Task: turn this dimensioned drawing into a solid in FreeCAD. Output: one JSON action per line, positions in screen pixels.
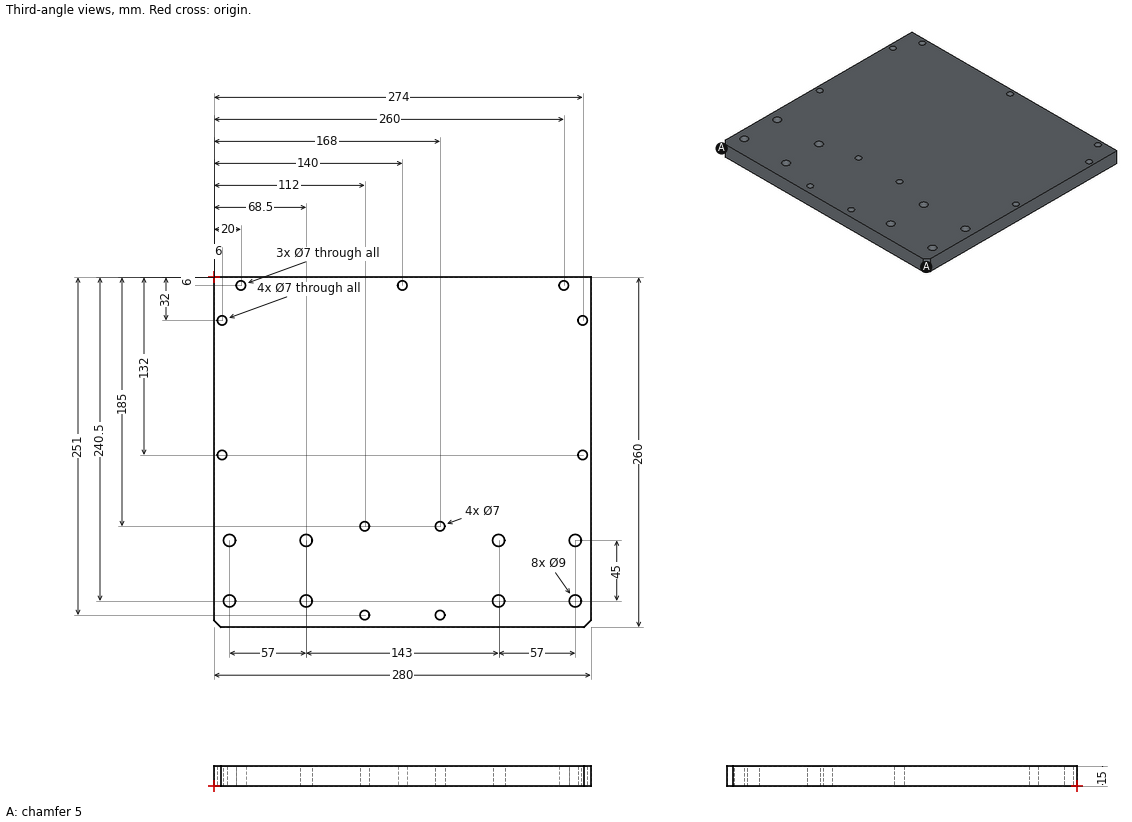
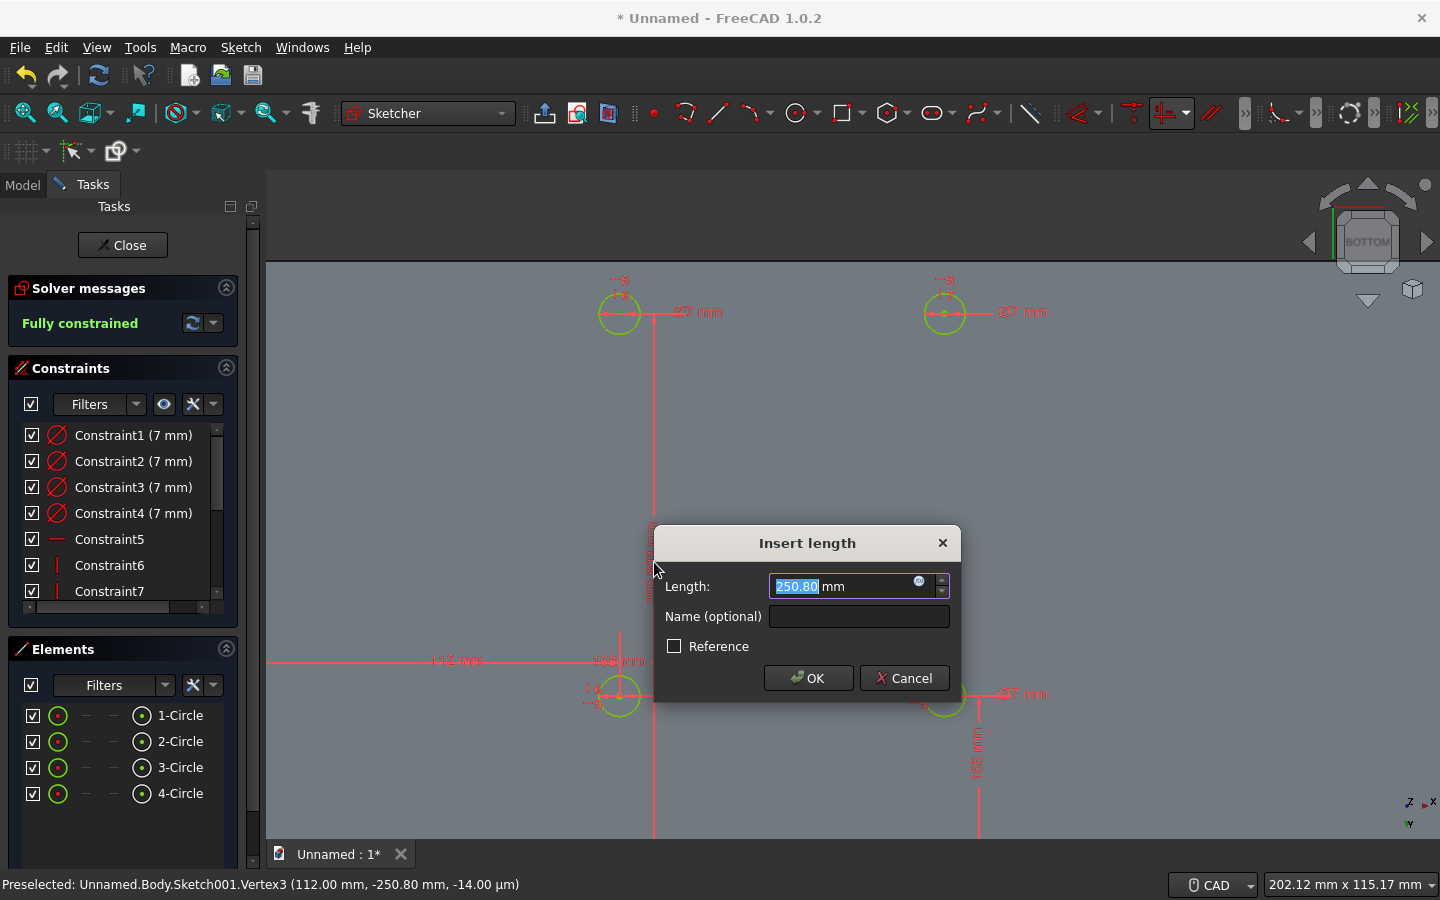
{"action": "type", "text": "251"}
{"action": "key", "text": "Return"}
{"action": "key", "text": "Escape"}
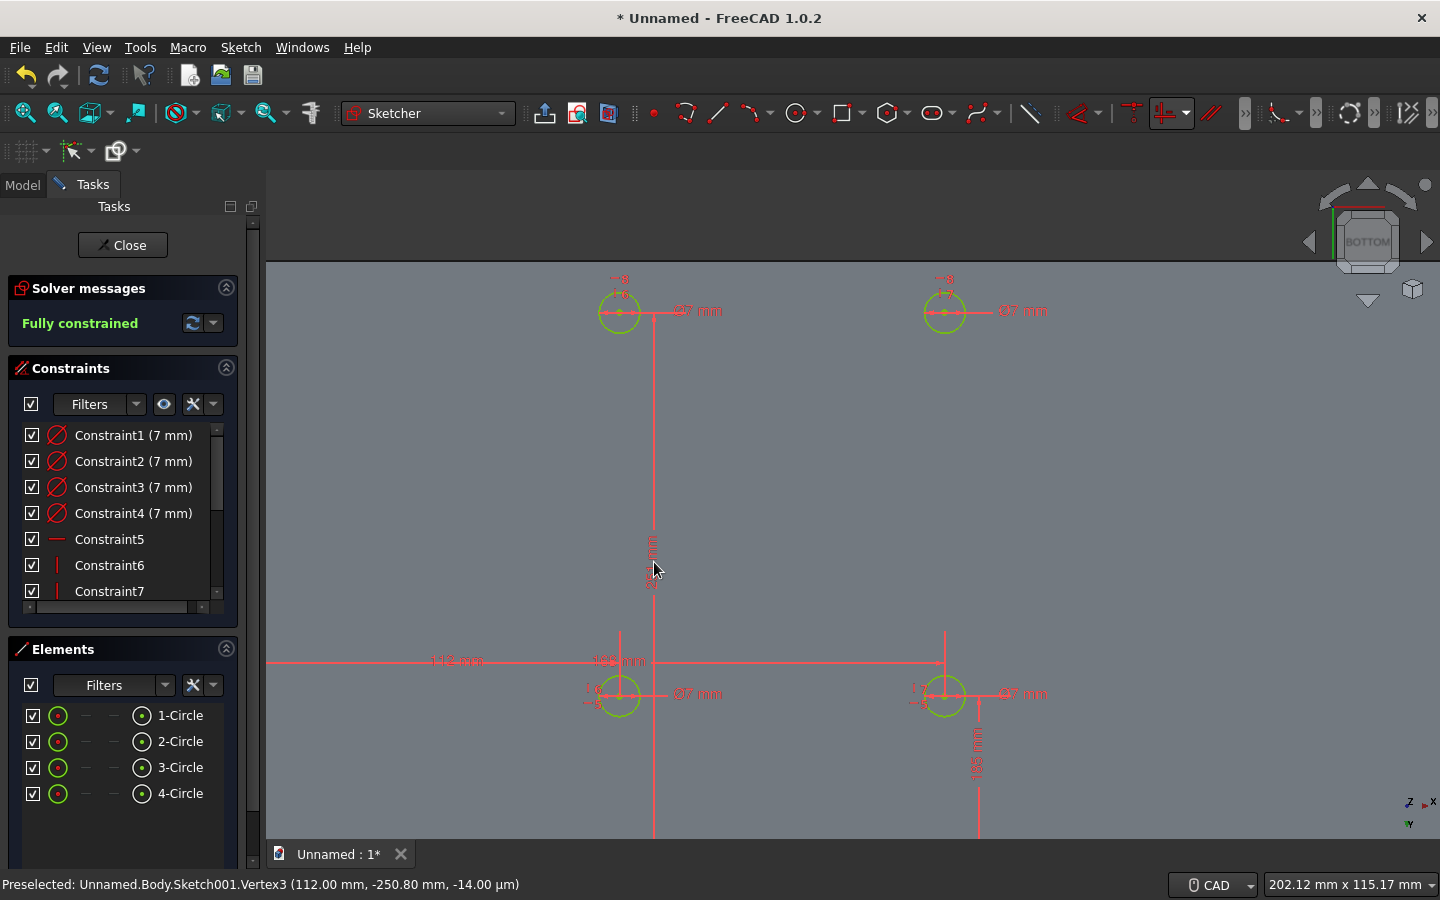
{"action": "left_click", "coordinate": [123, 245]}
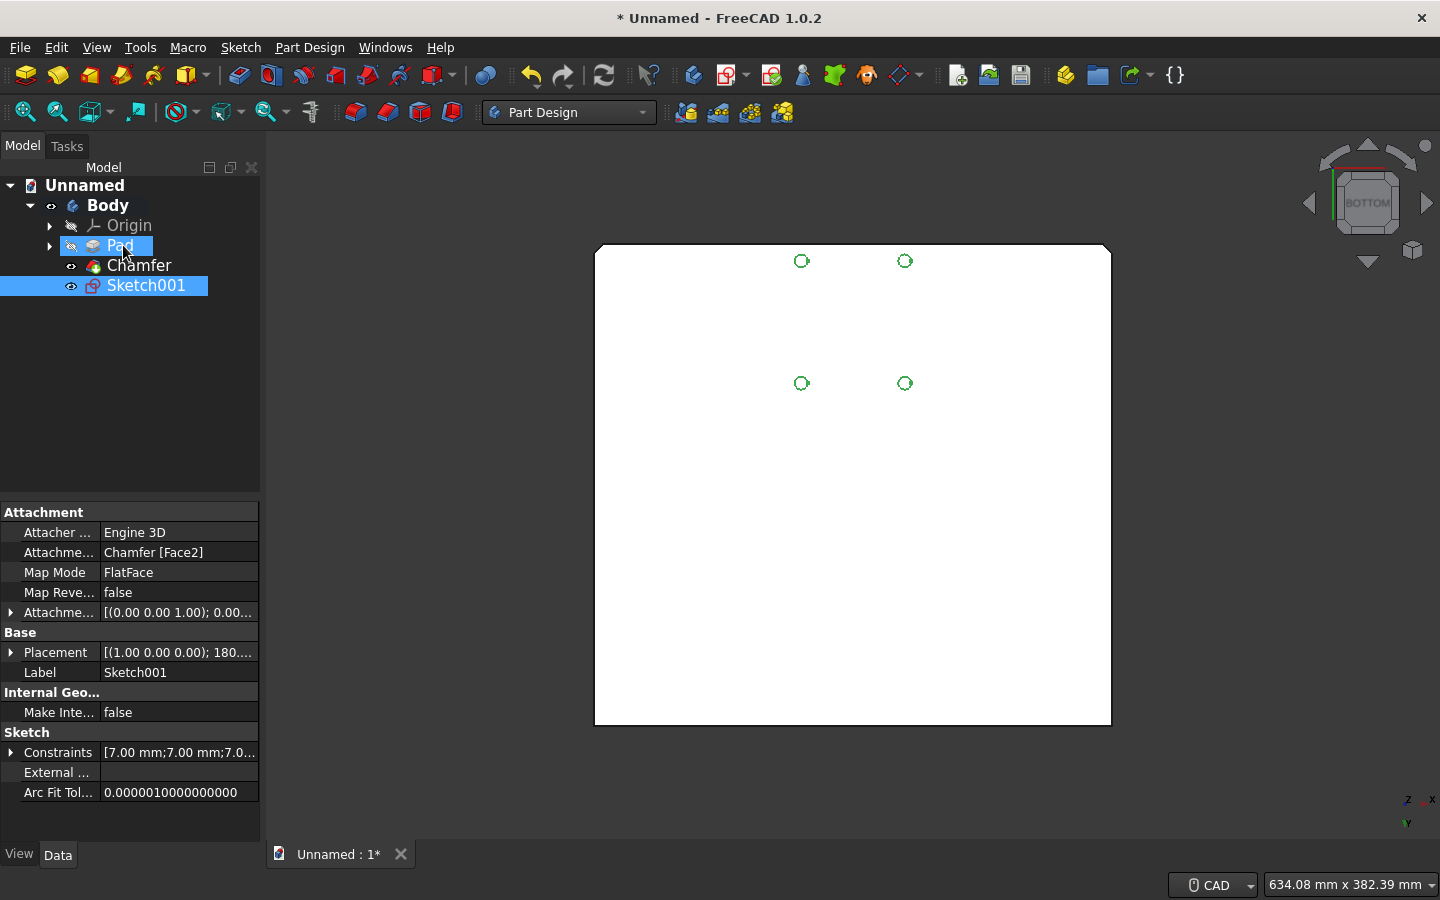
{"action": "left_click", "coordinate": [240, 76]}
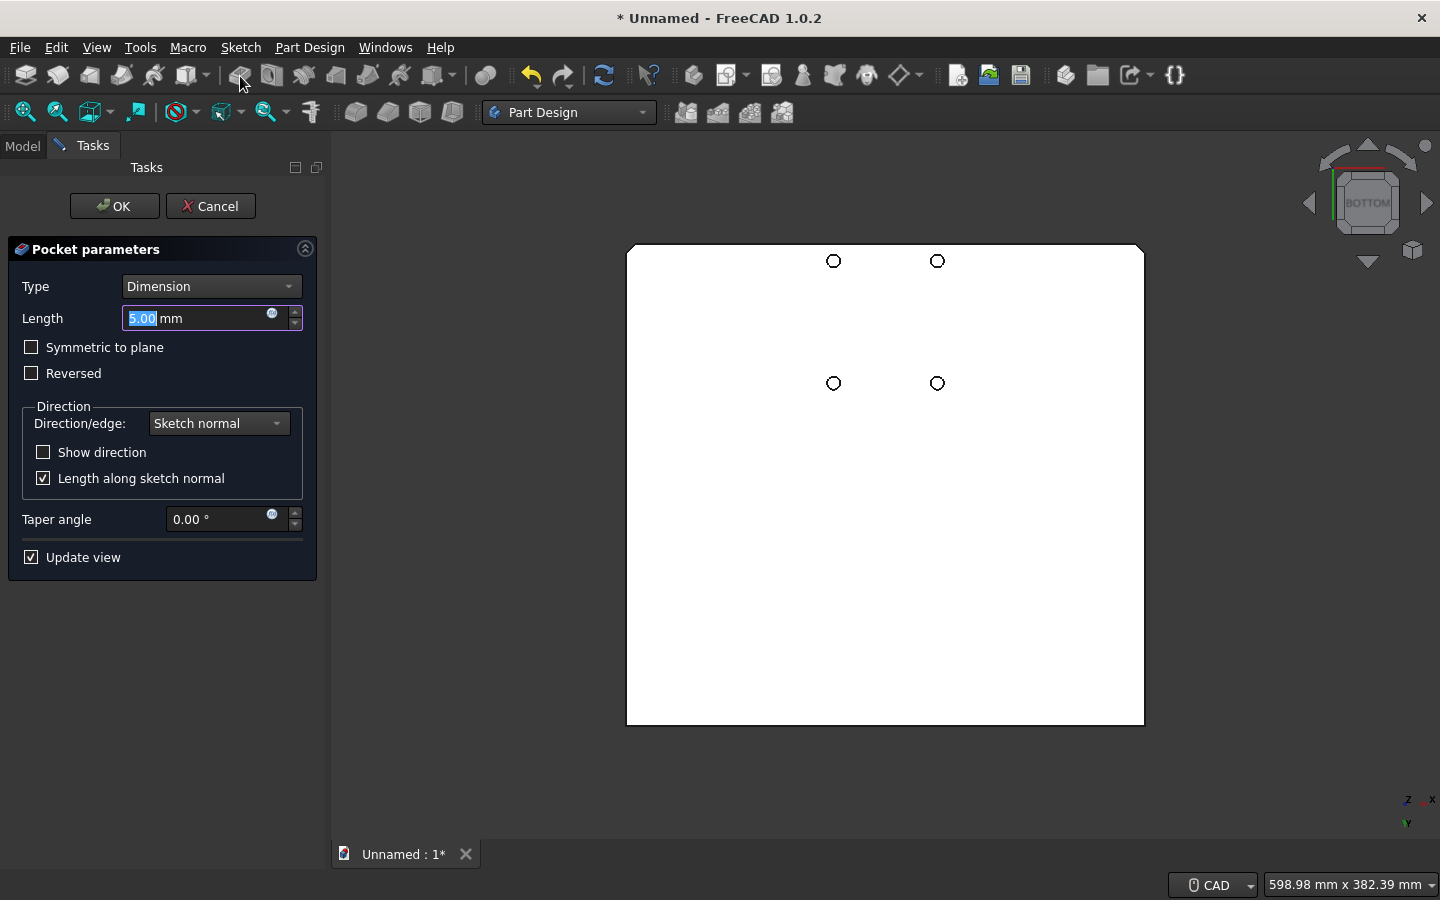
{"action": "left_click", "coordinate": [212, 286]}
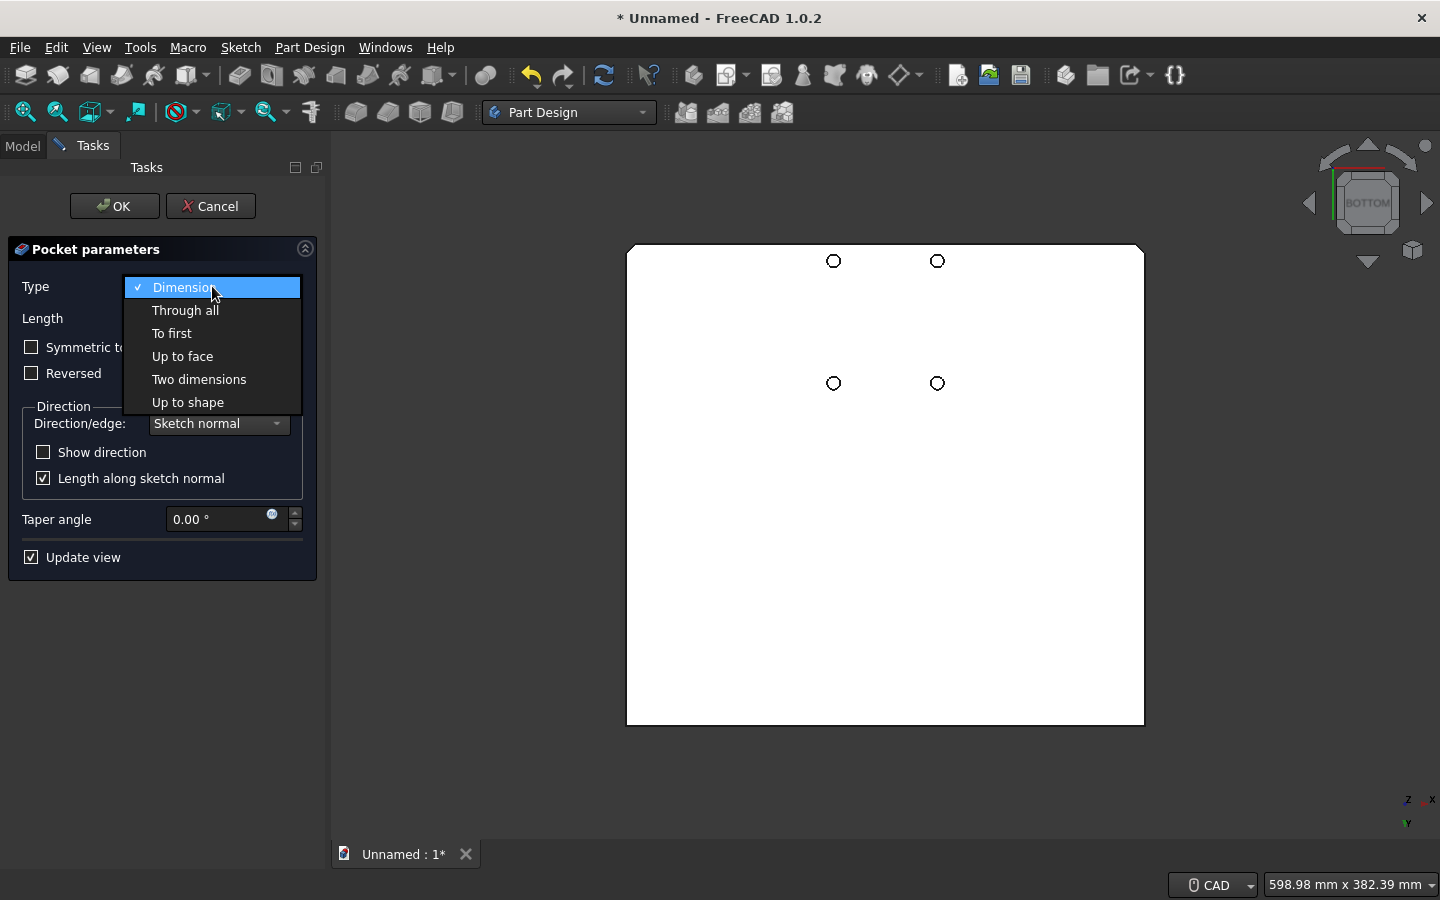
{"action": "left_click", "coordinate": [212, 310]}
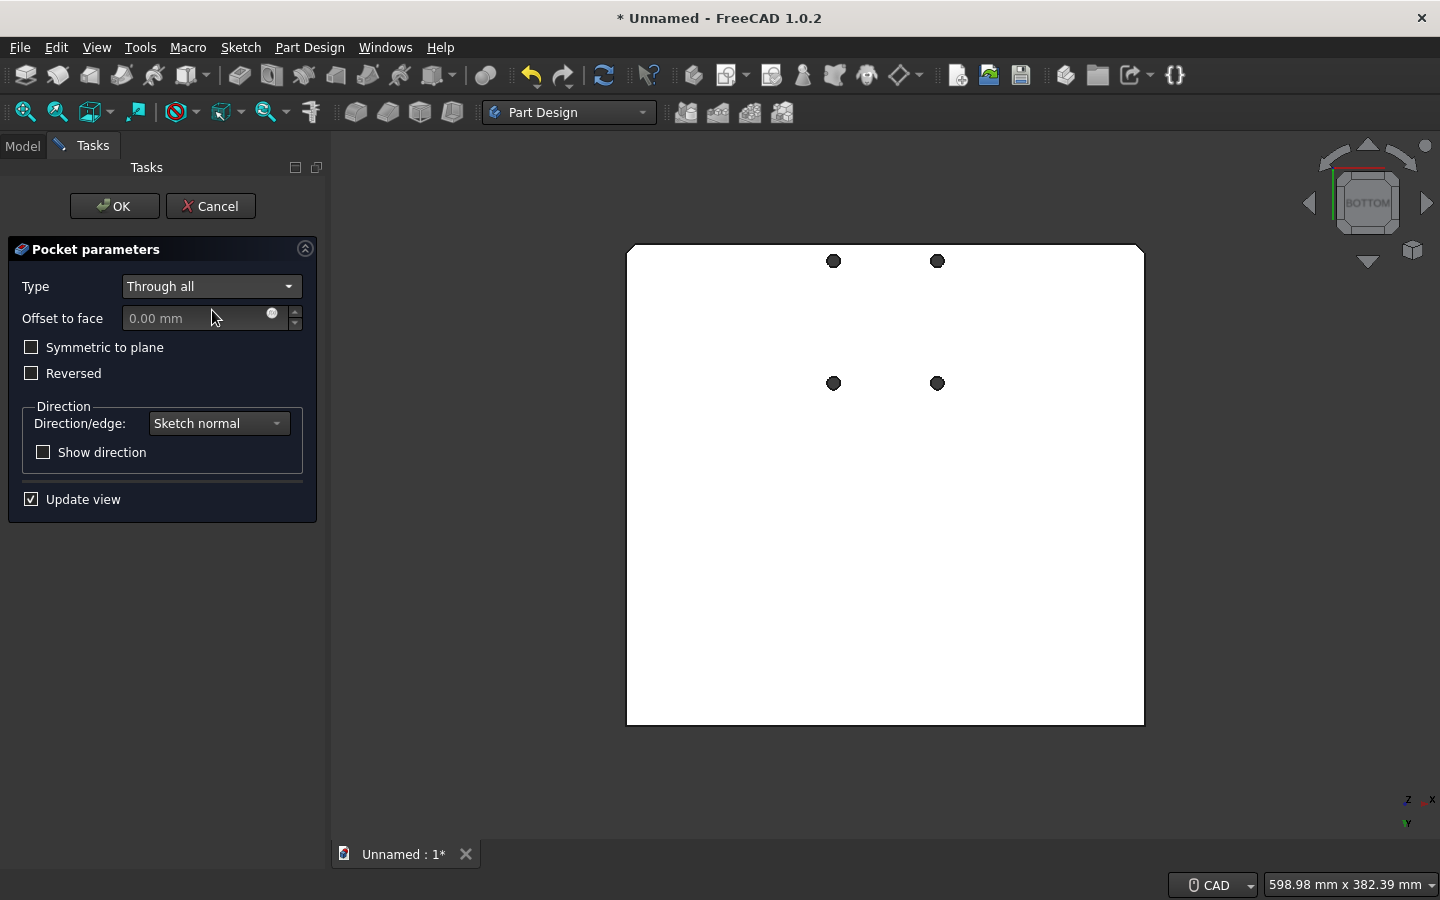
{"action": "left_click", "coordinate": [115, 206]}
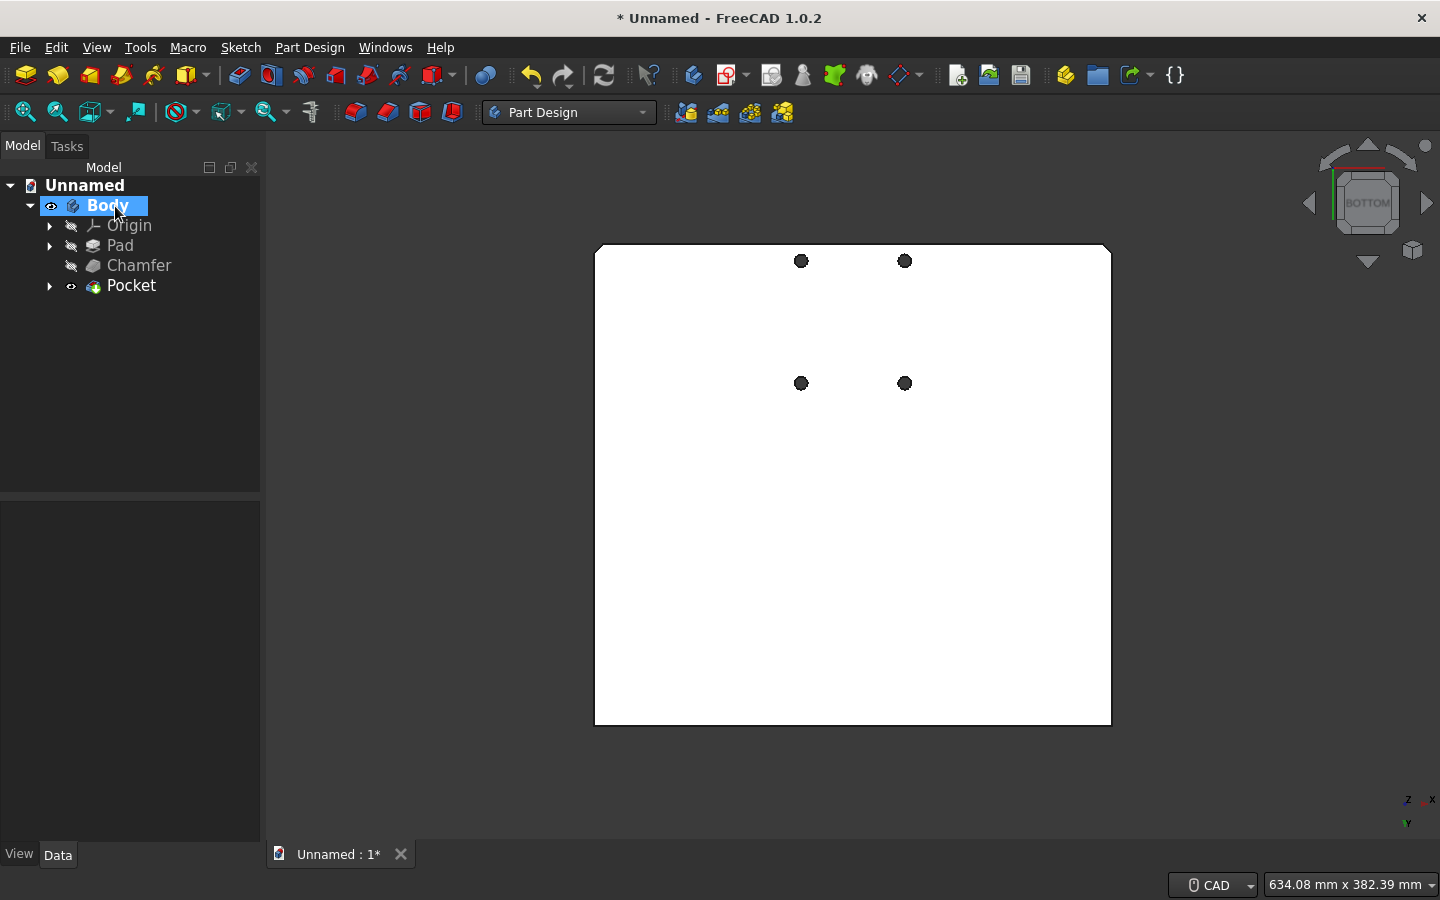
{"action": "key", "text": "0"}